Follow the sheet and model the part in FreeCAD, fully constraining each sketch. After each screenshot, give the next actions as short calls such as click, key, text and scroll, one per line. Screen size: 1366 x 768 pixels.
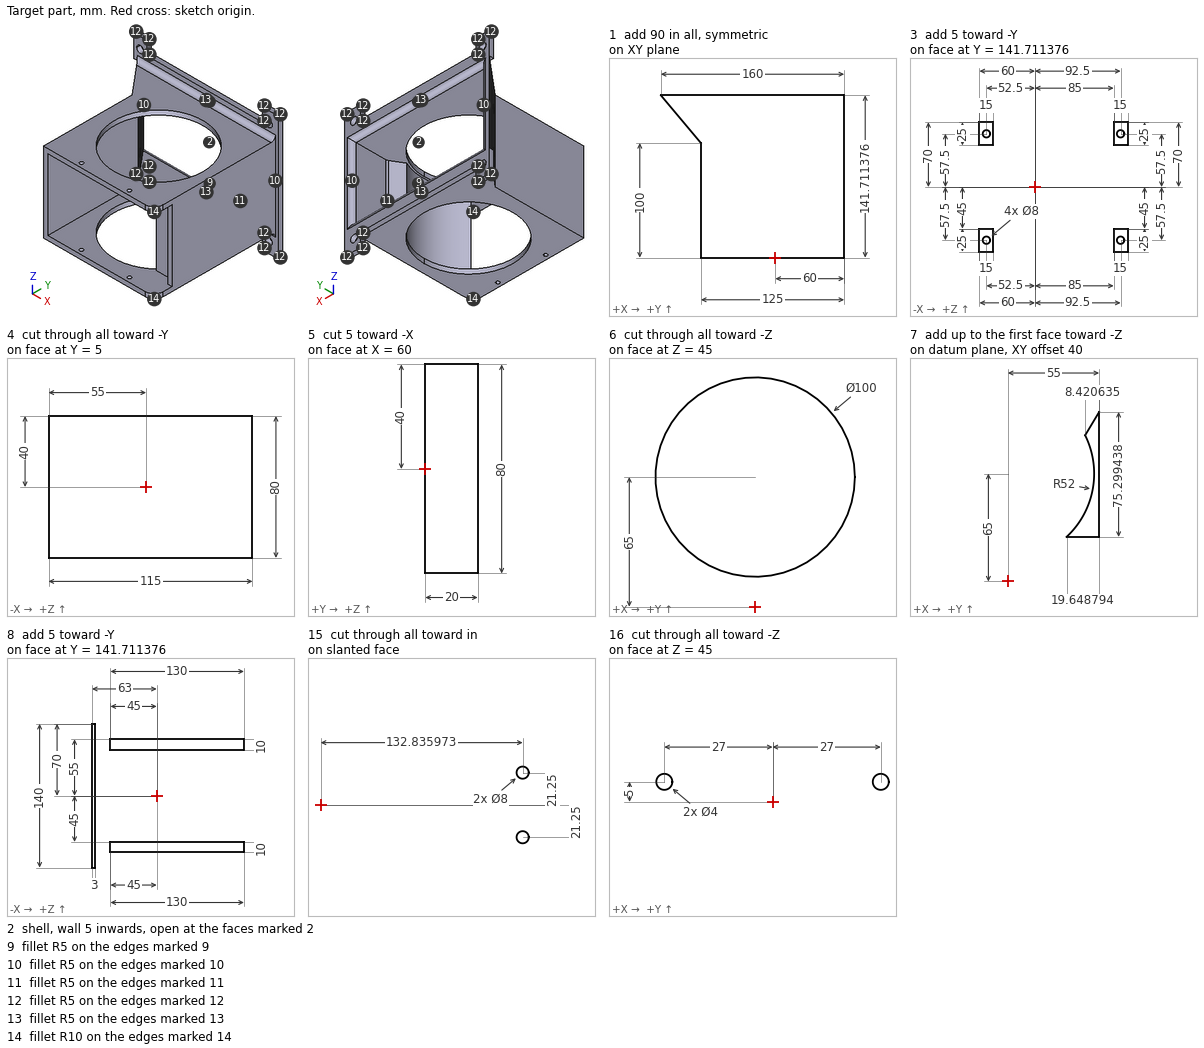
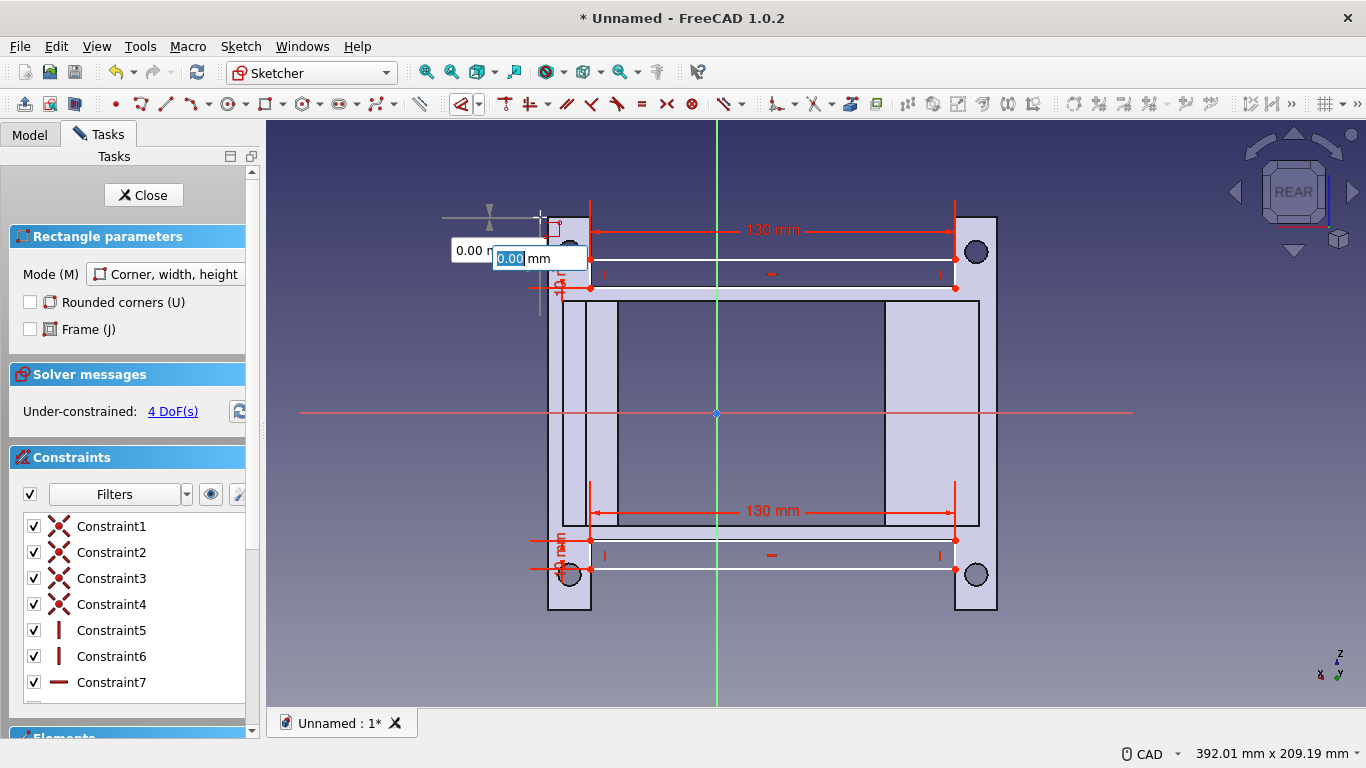
click(548, 610)
key(Escape)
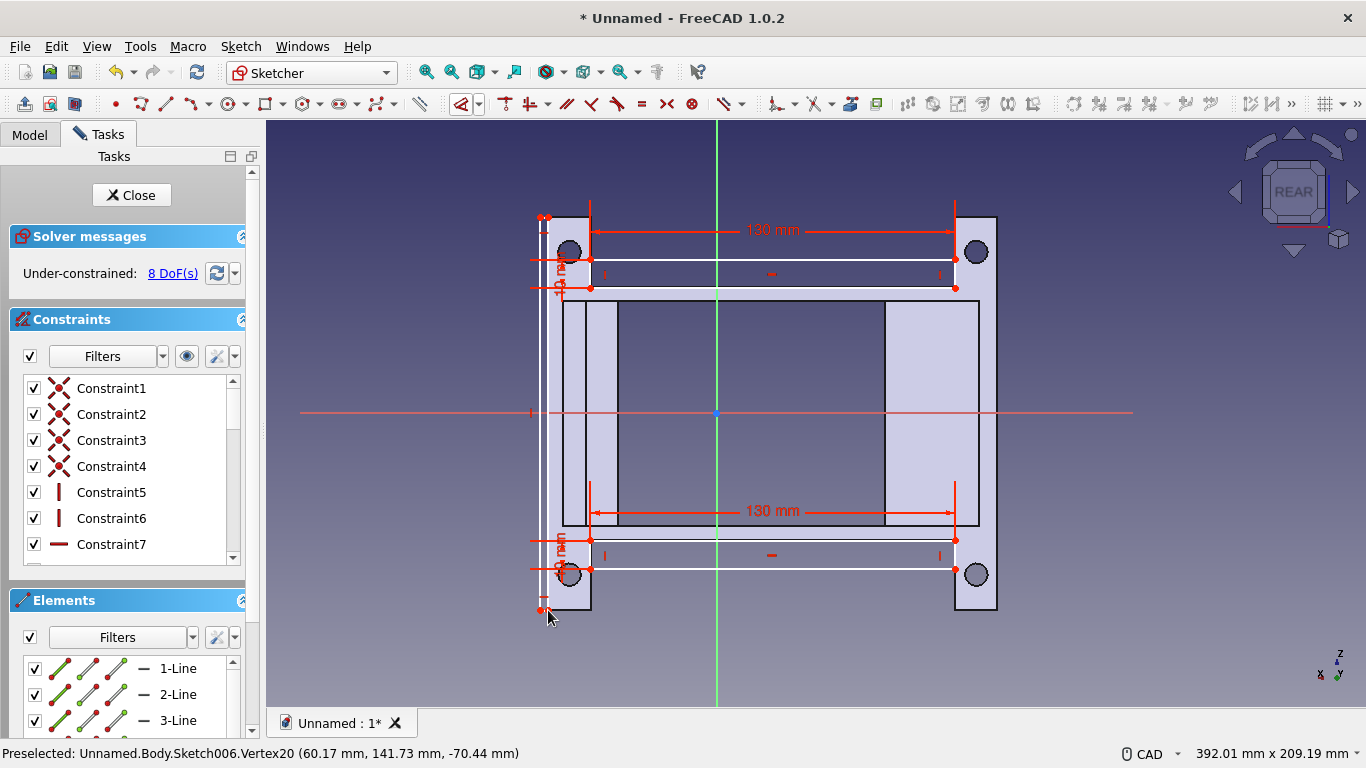
scroll(544, 611, up, 8)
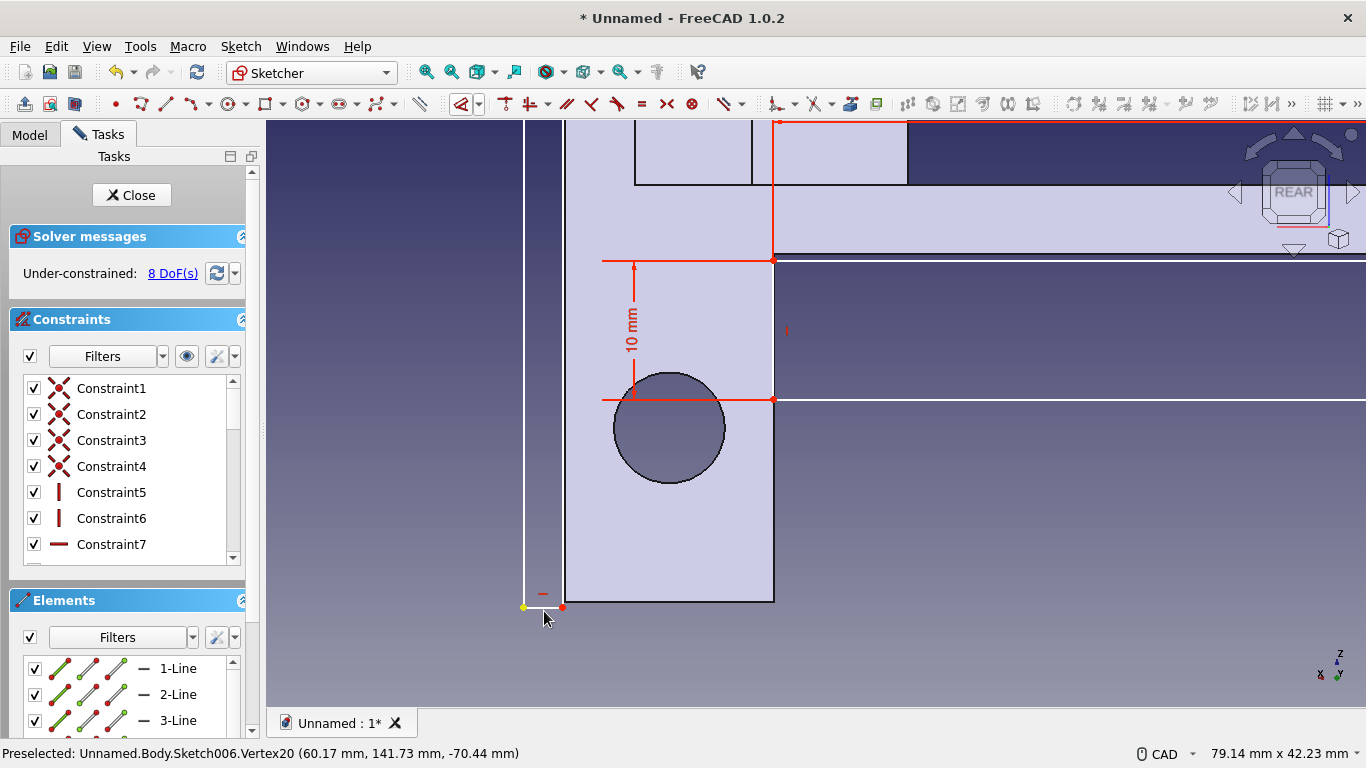
click(543, 608)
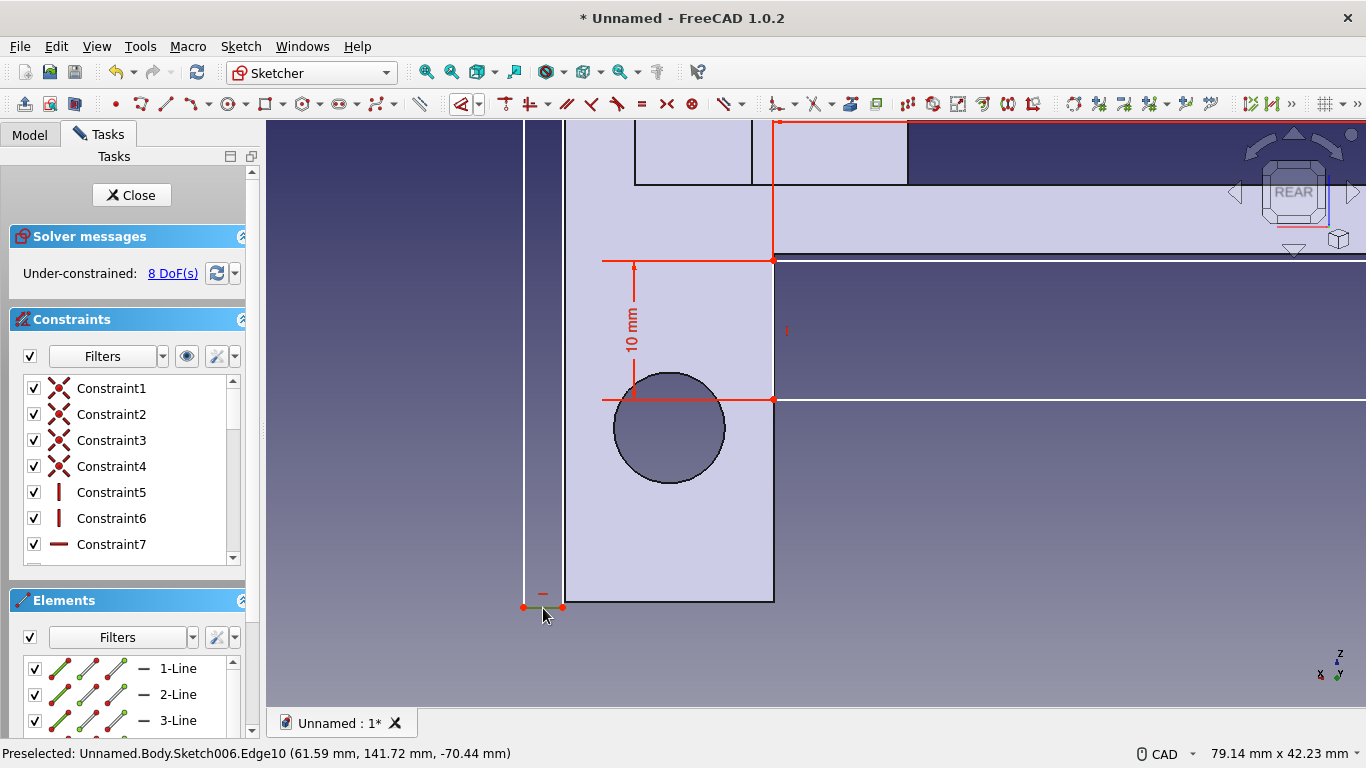
key(l)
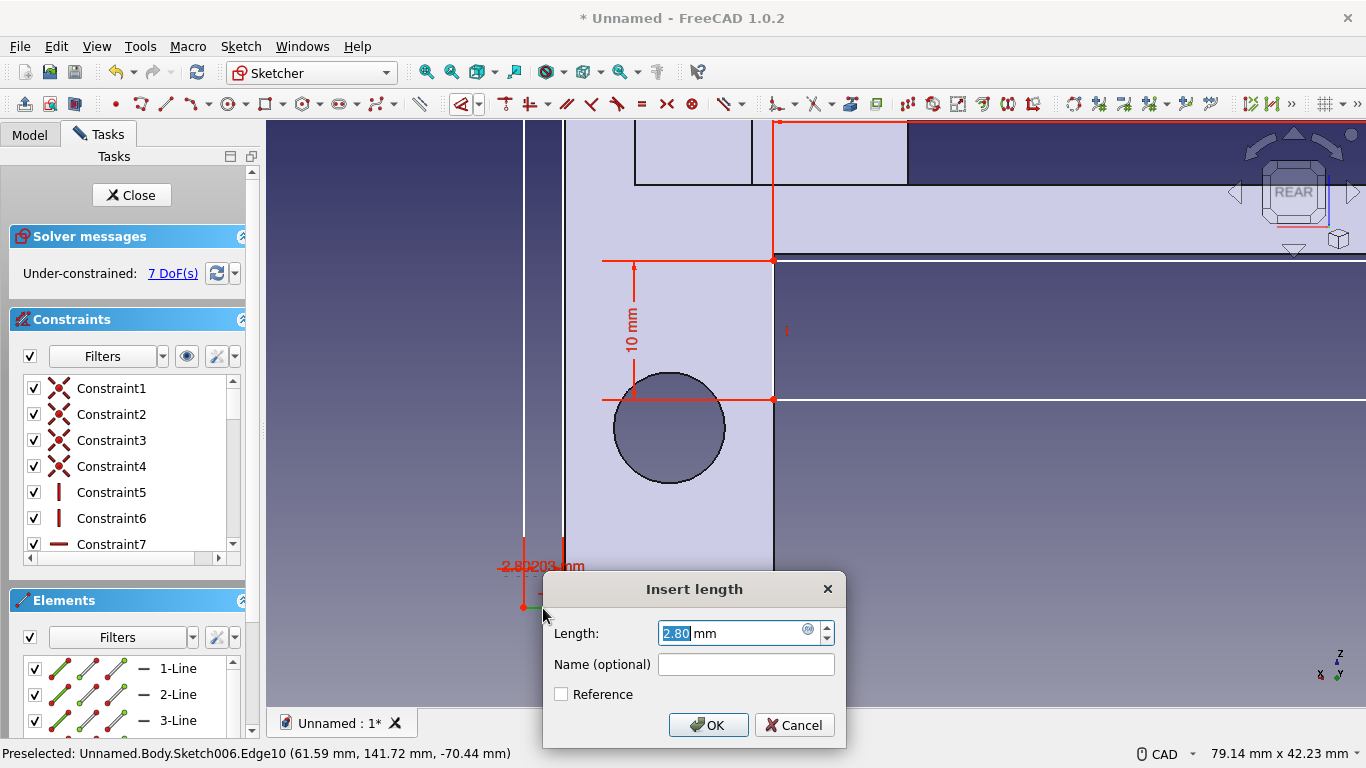
text(3)
key(Return)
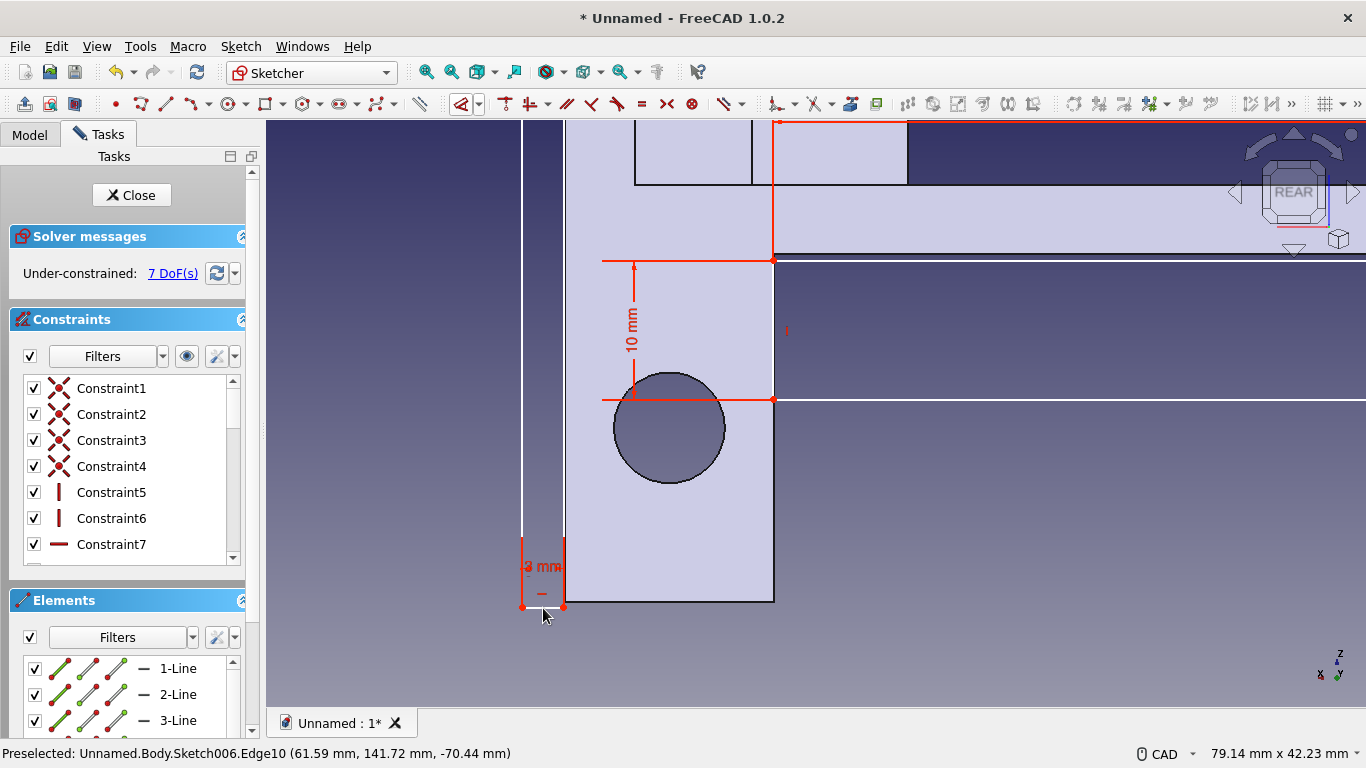
scroll(544, 612, down, 8)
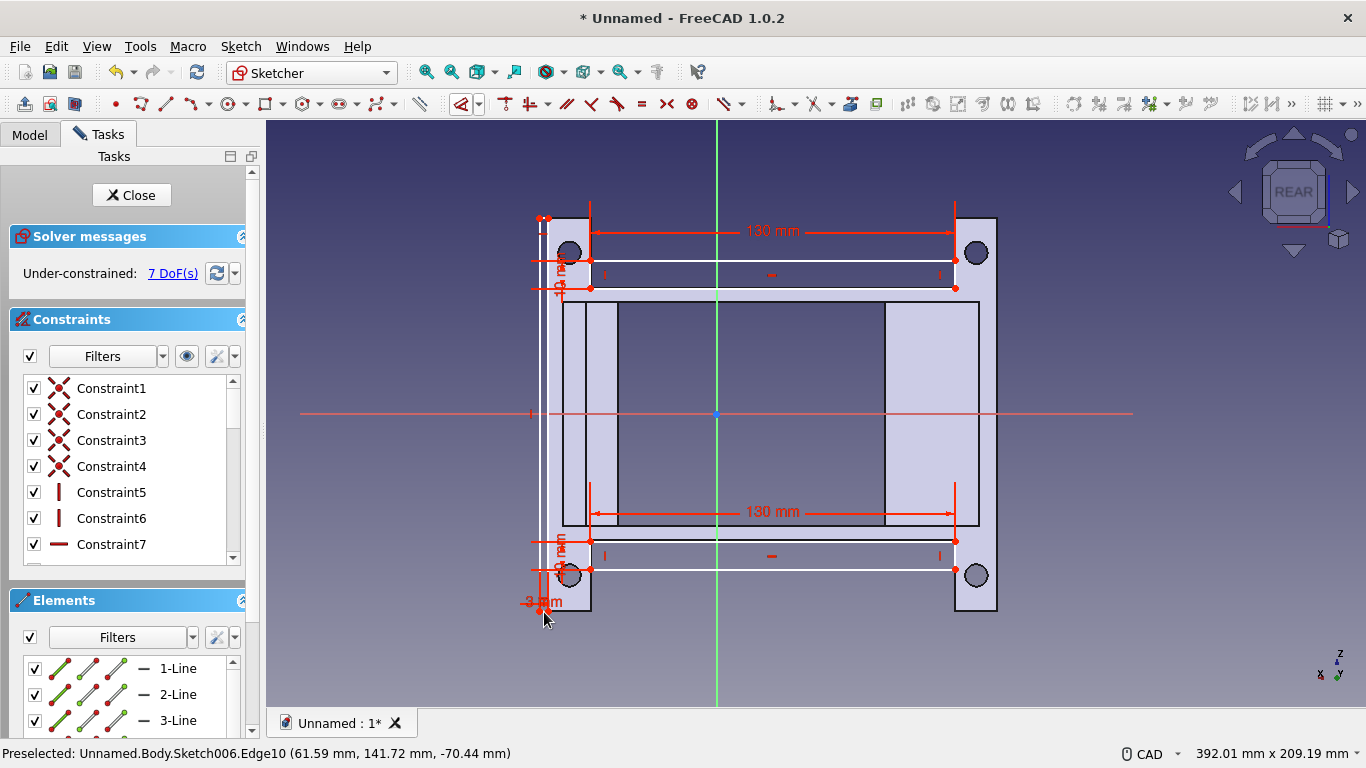
scroll(540, 533, up, 3)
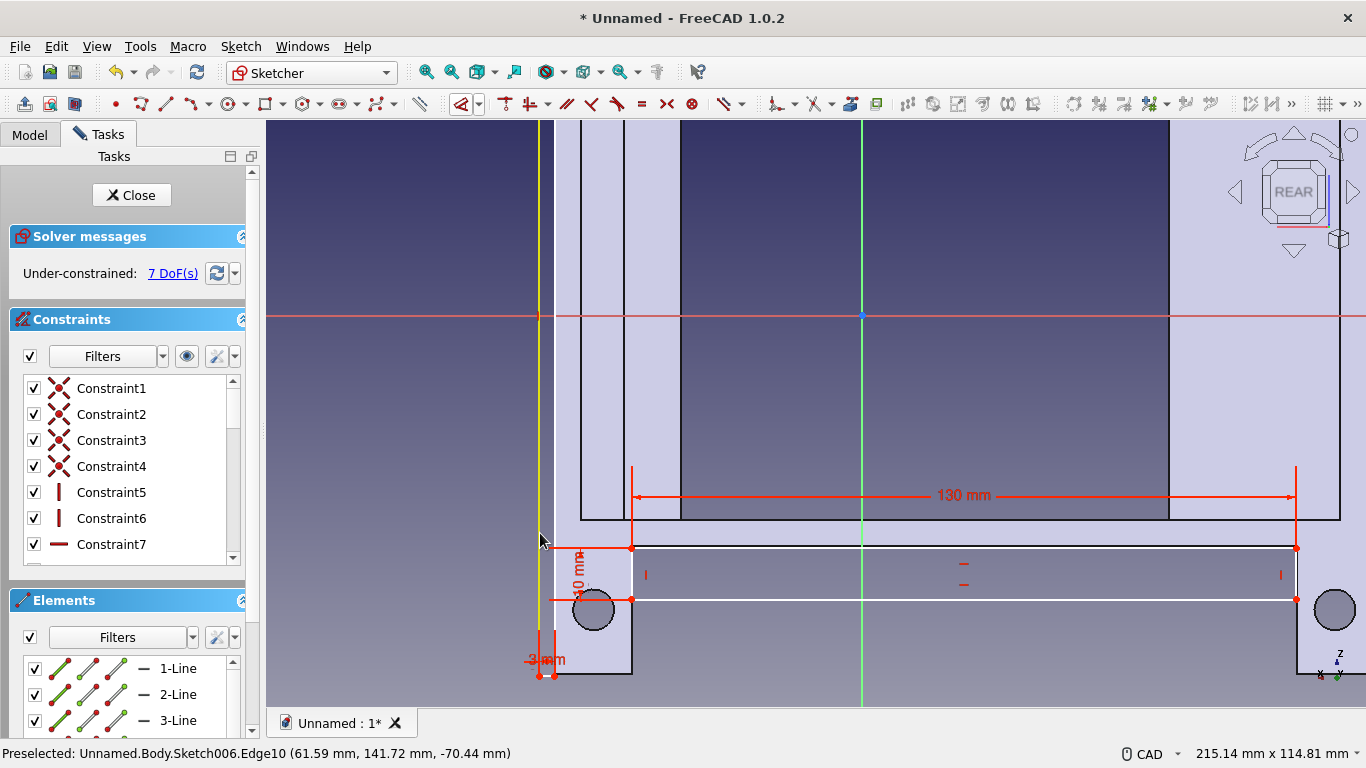
click(539, 533)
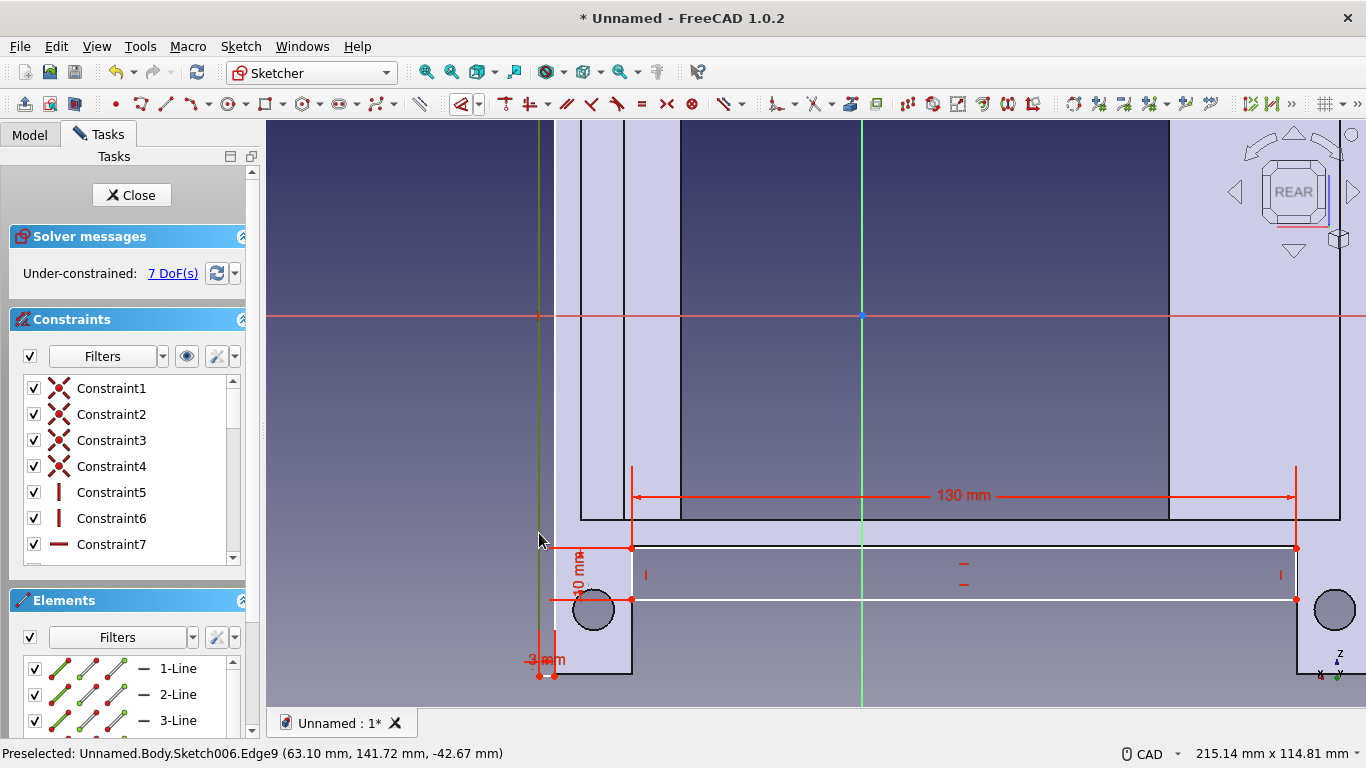
click(478, 104)